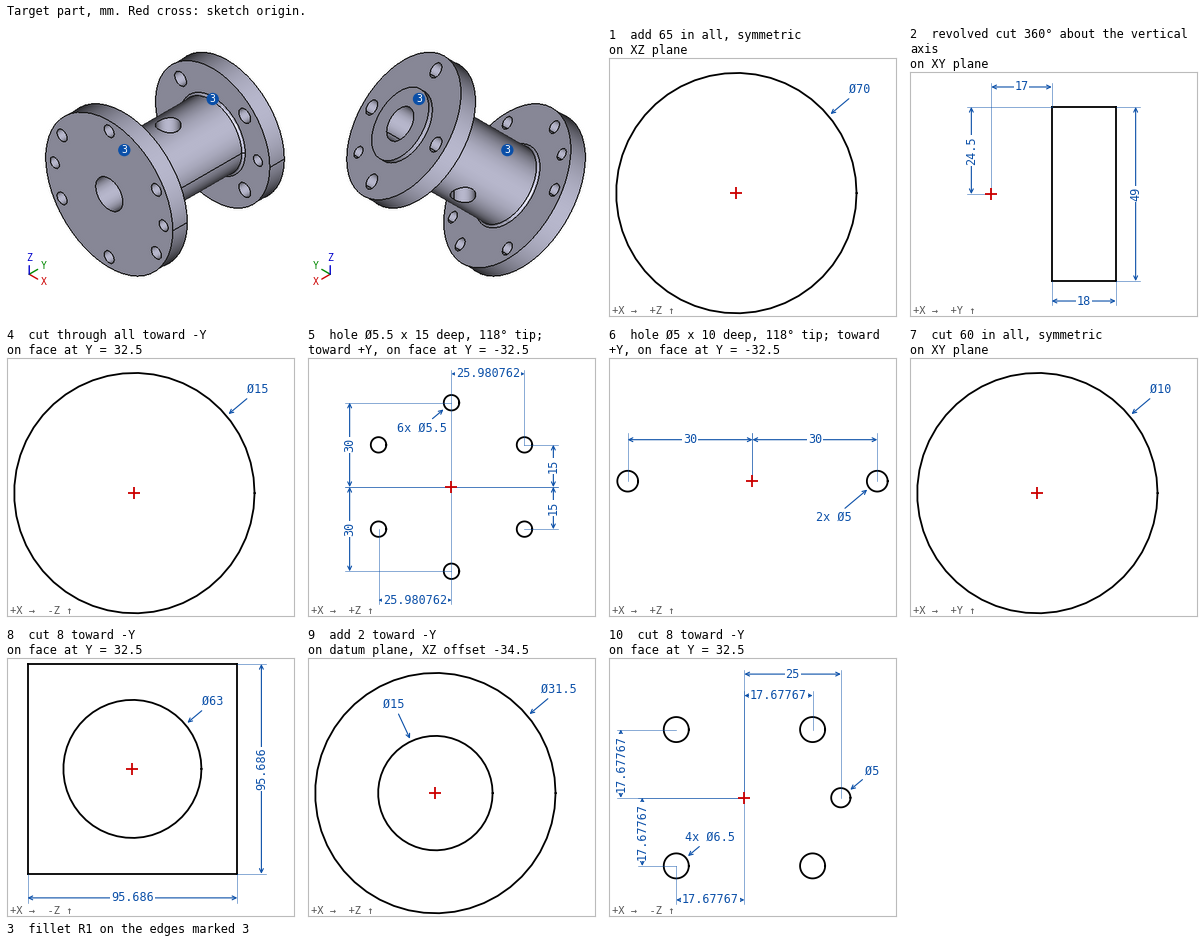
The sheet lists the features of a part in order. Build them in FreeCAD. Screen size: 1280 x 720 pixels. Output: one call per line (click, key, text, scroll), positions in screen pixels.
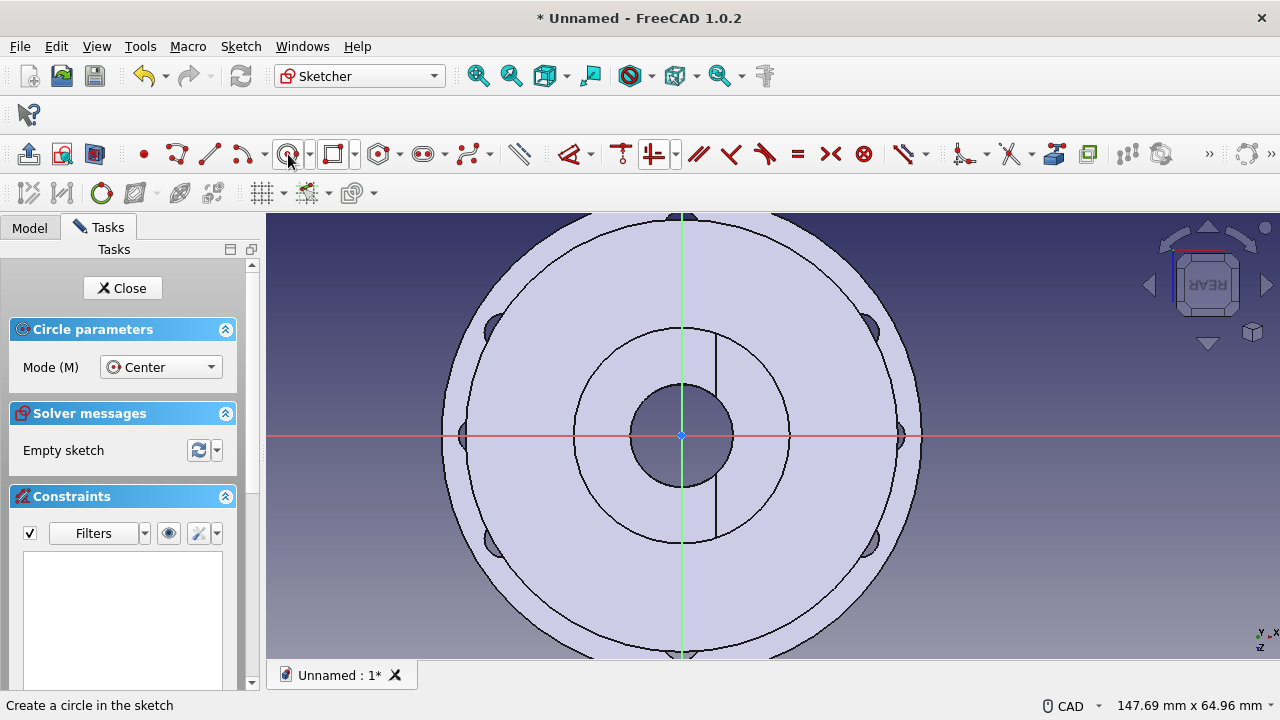
click(560, 557)
move(576, 541)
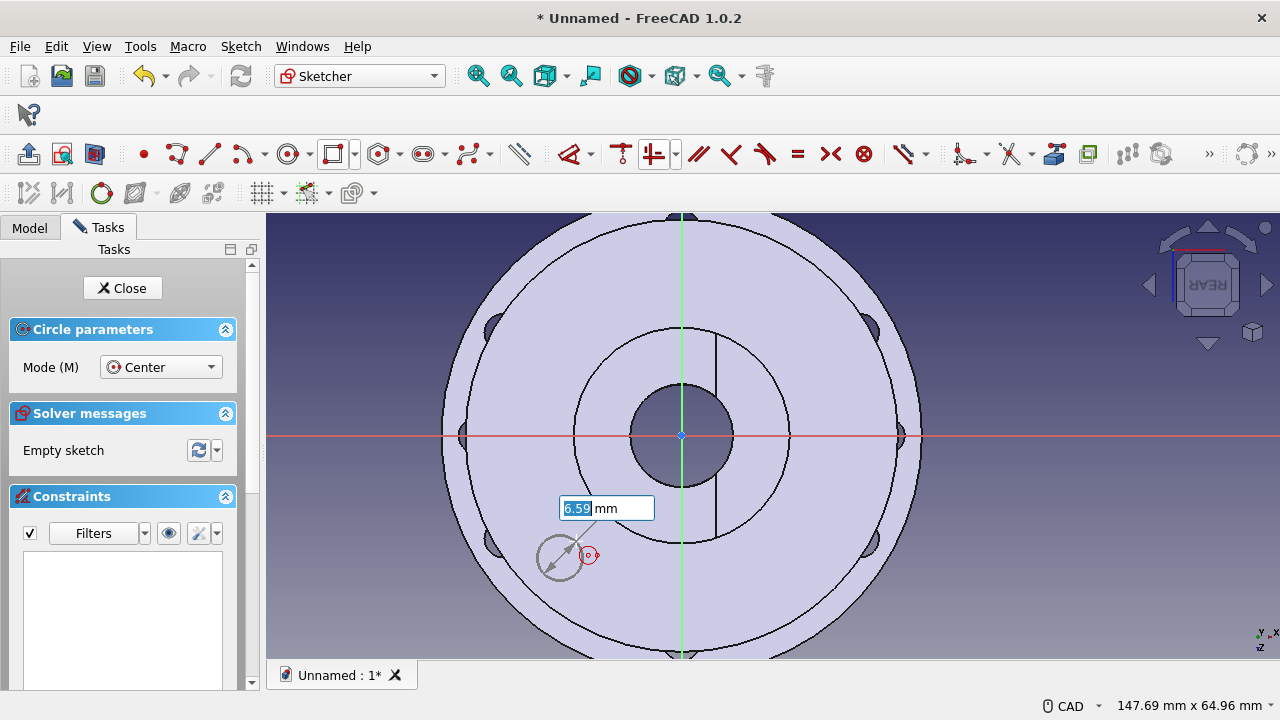
text(6.5)
key(Return)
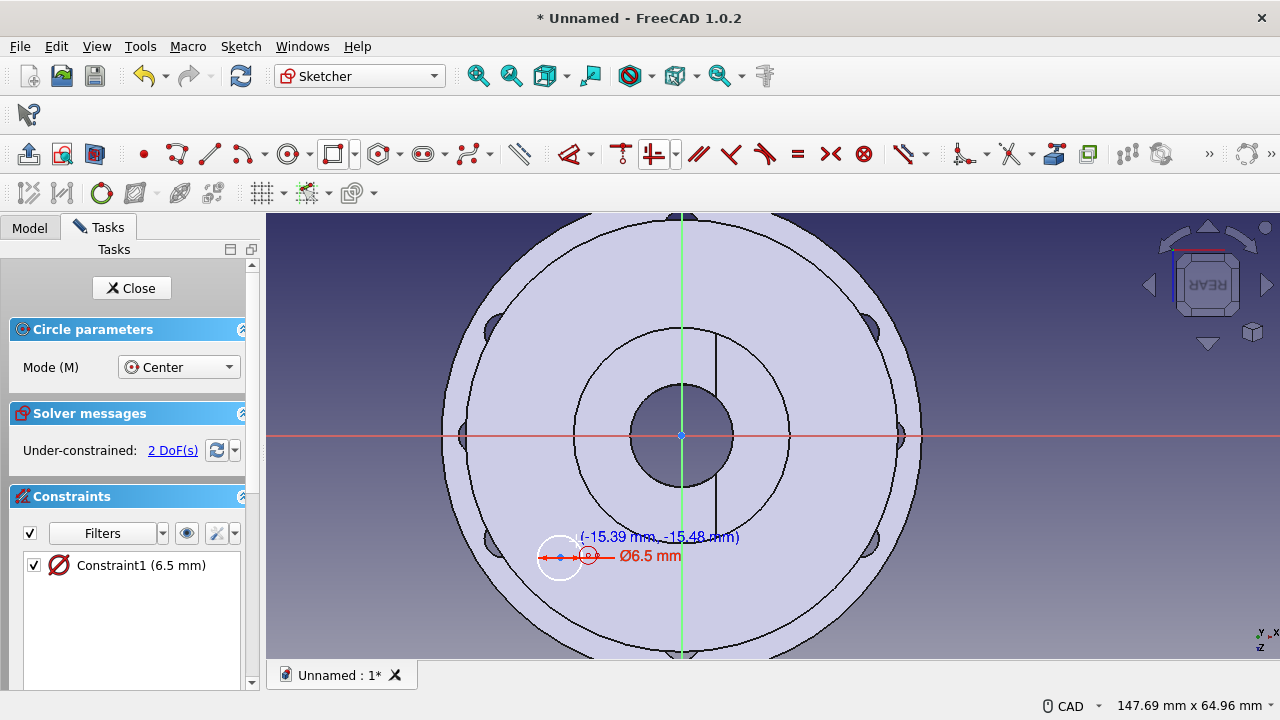
click(560, 314)
move(576, 299)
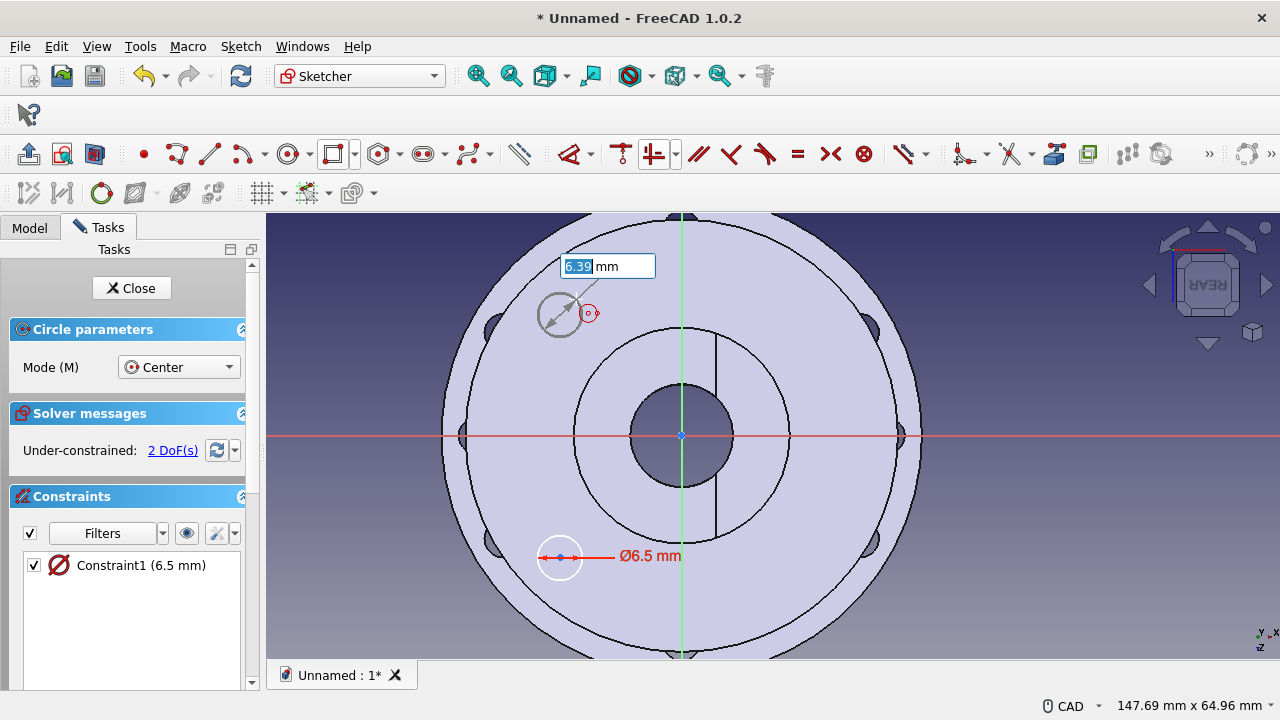
text(6.5)
key(Return)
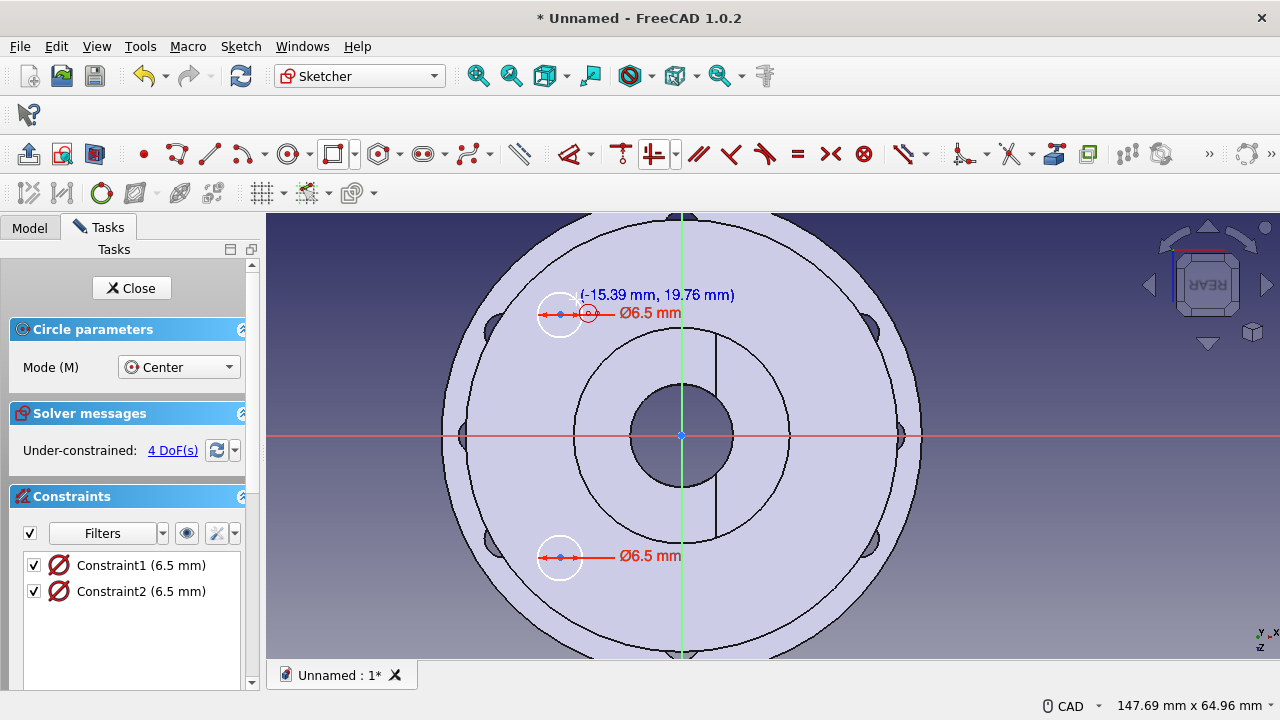
click(803, 314)
move(819, 299)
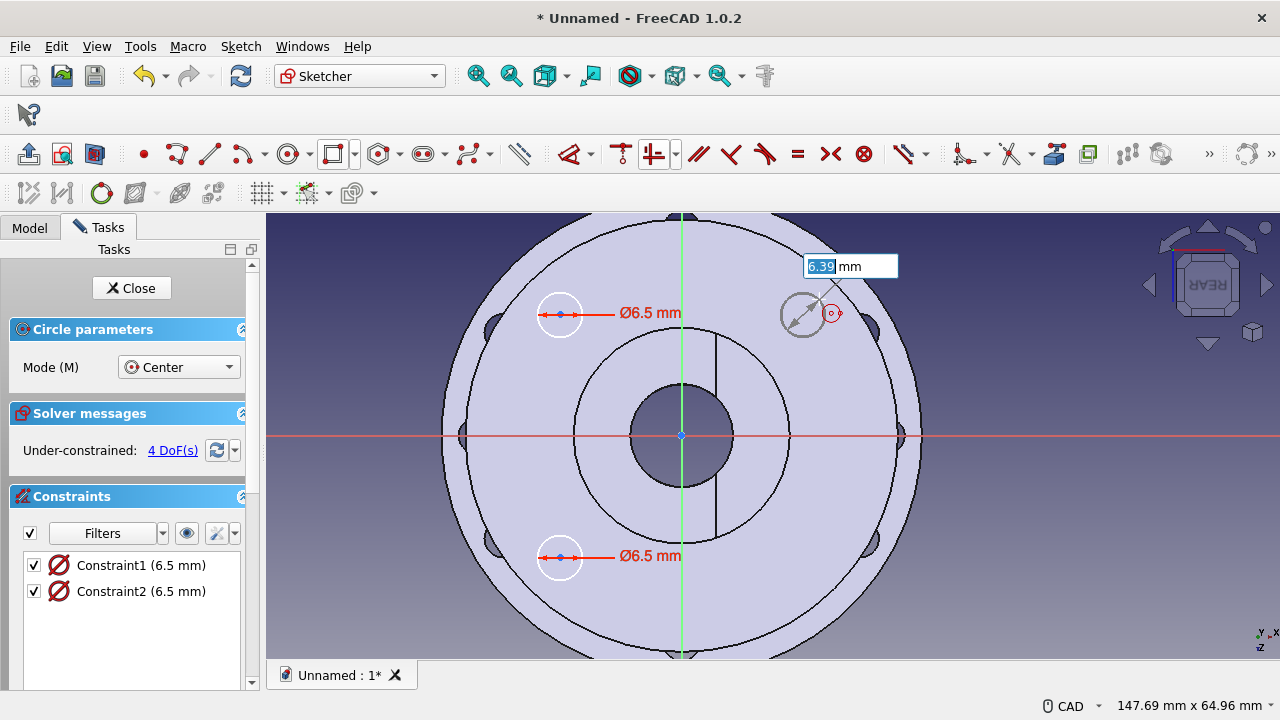
text(6.5)
key(Return)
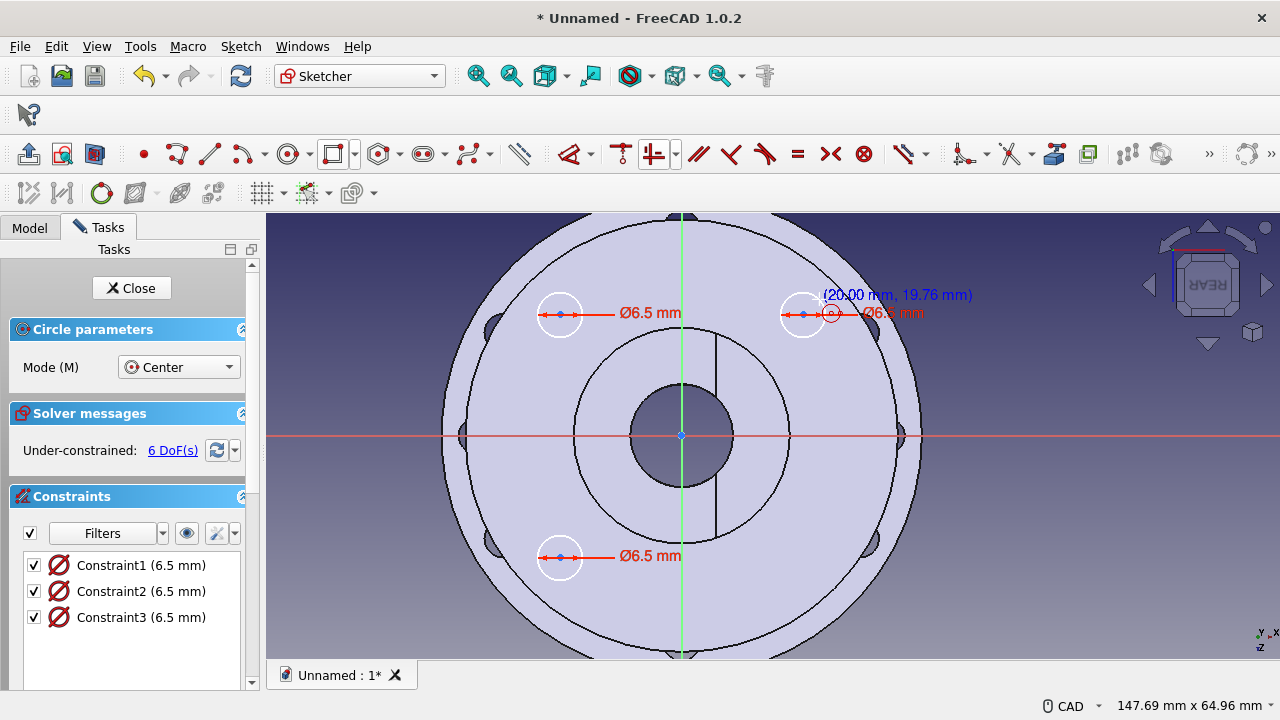
click(803, 557)
move(819, 541)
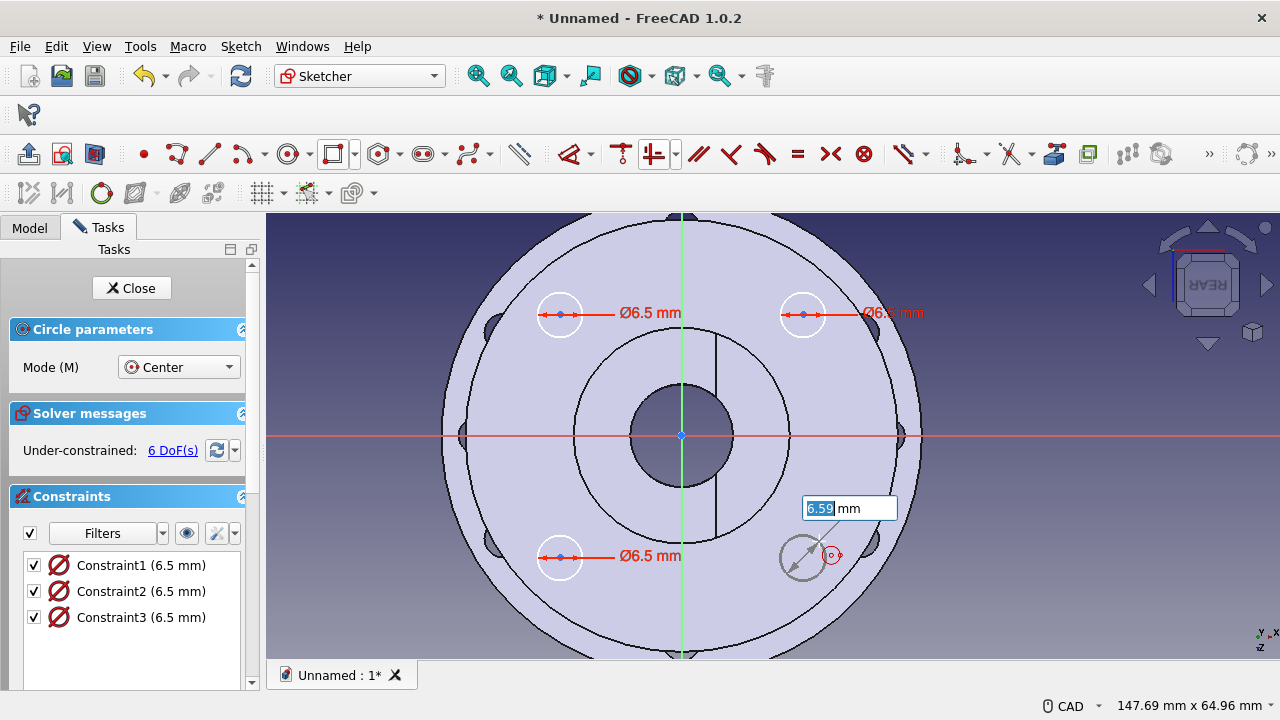
text(6.5)
key(Return)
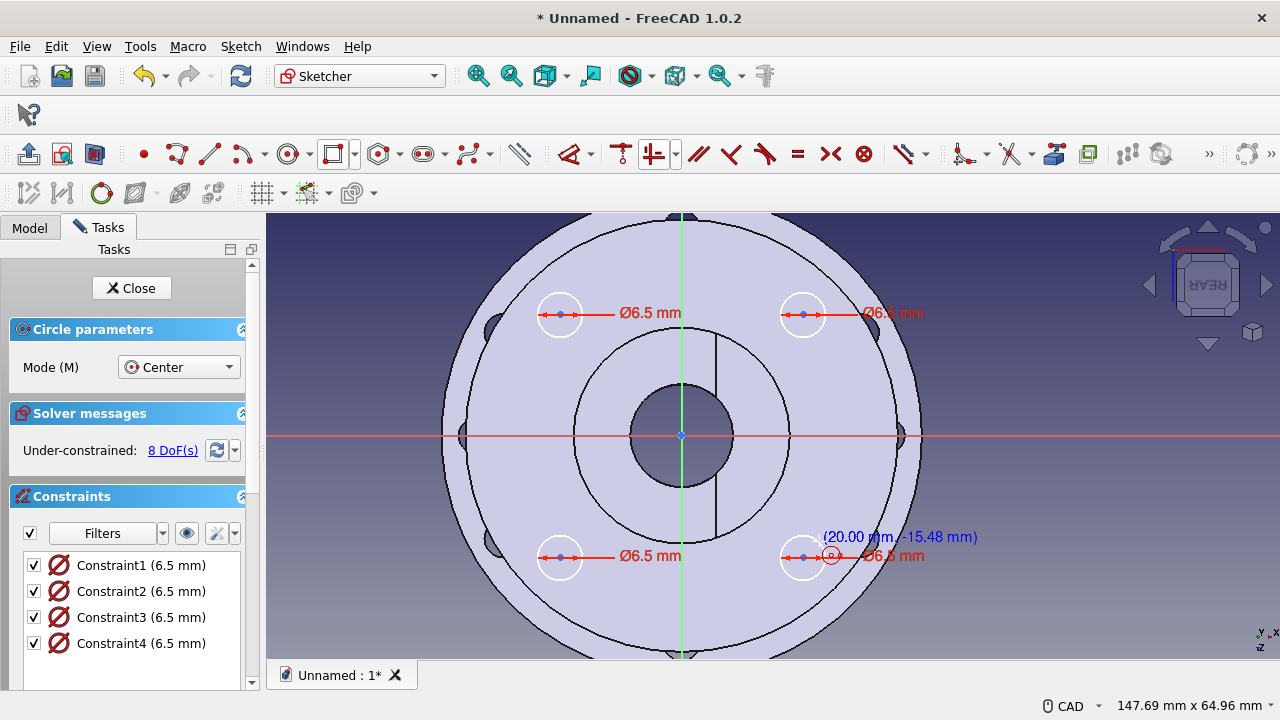
scroll(853, 436, up, 2)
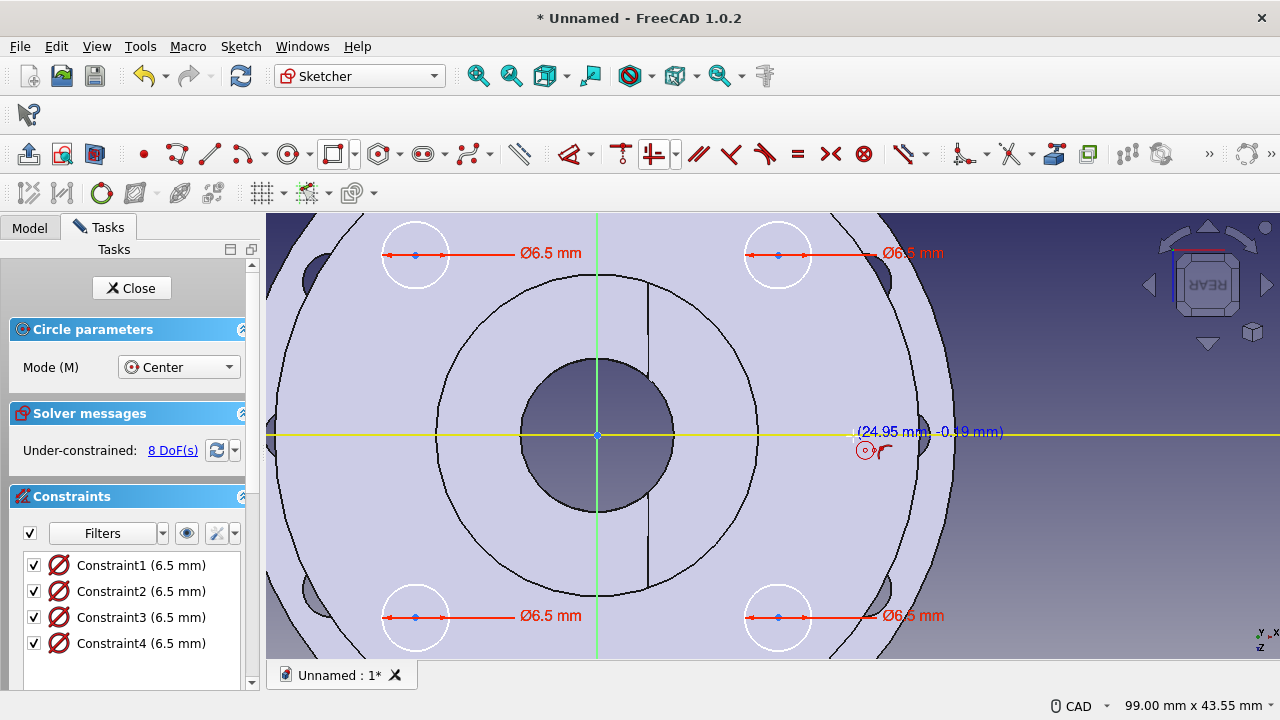
click(853, 435)
move(871, 417)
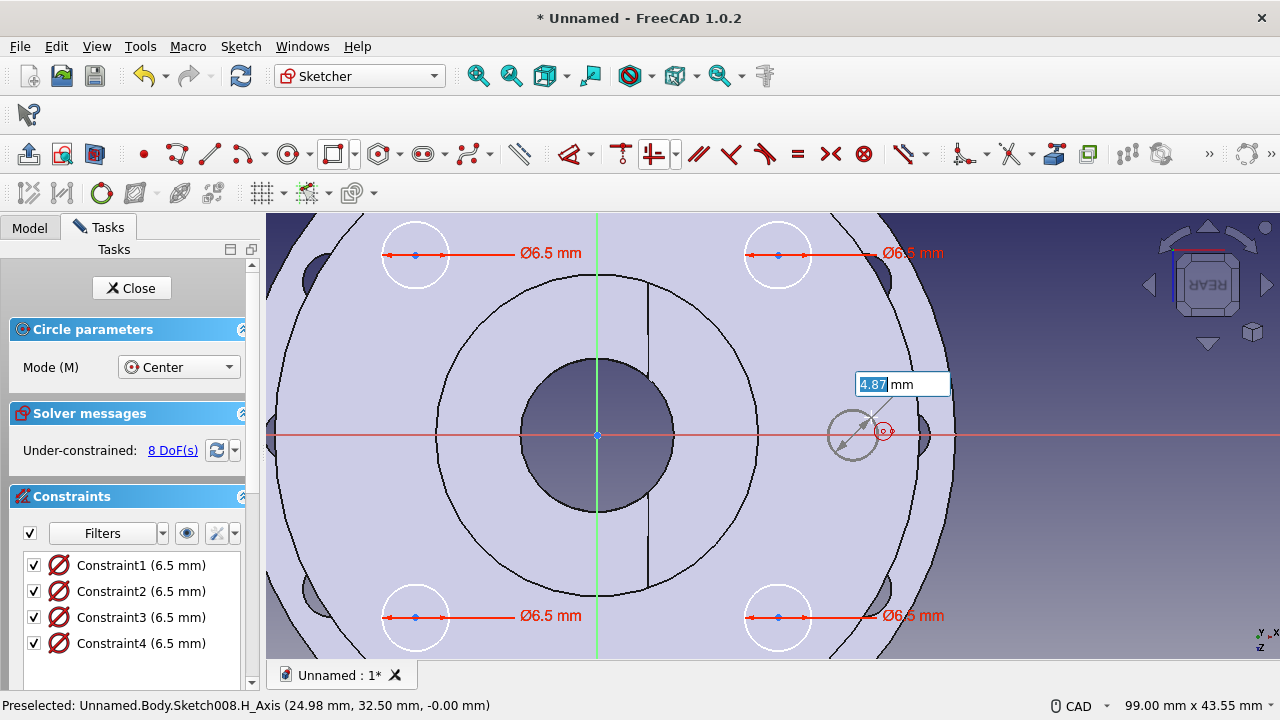
text(5)
key(Return)
key(Escape)